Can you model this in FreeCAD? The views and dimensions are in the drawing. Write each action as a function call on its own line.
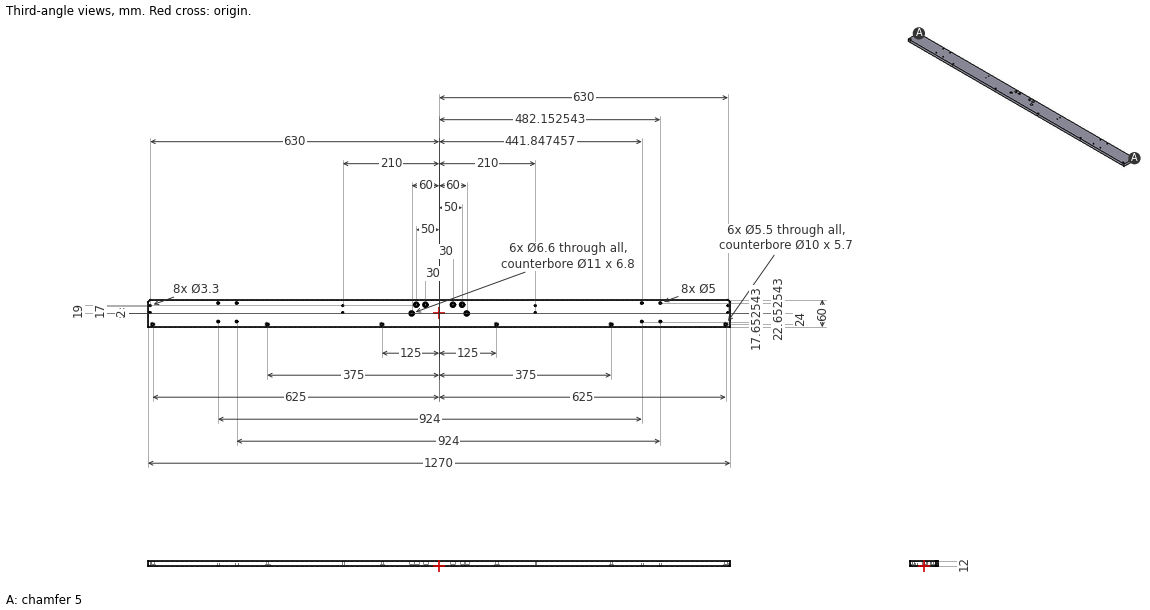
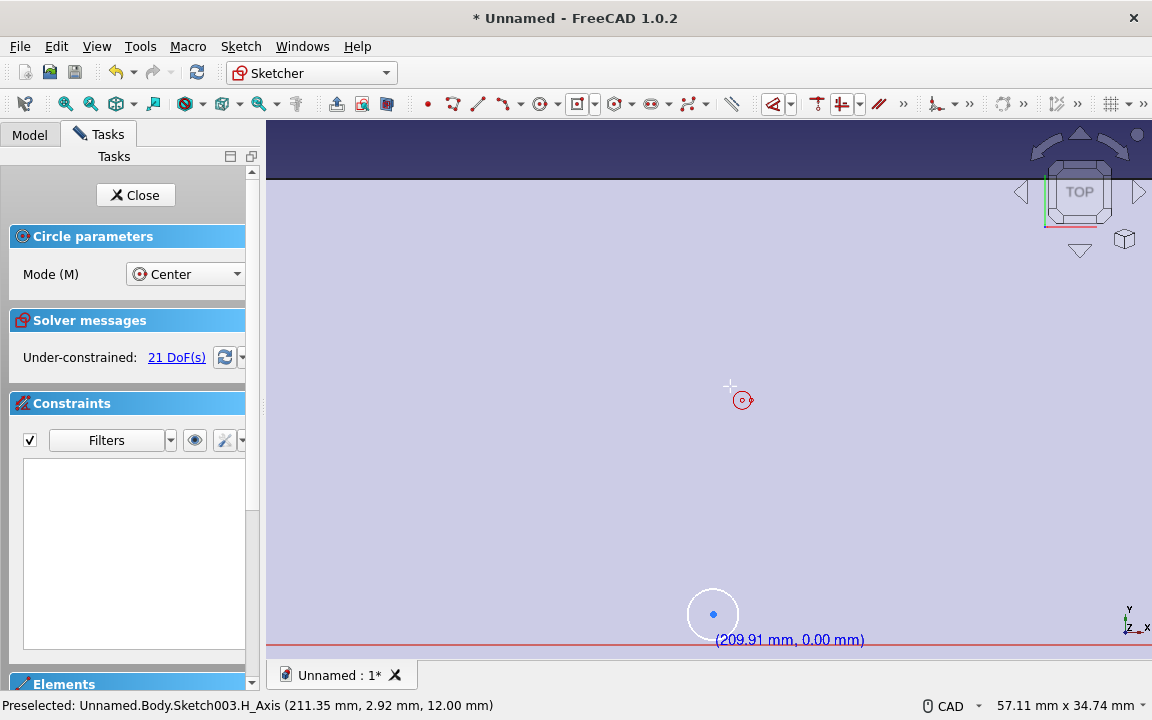
scroll(730, 386, down, 18)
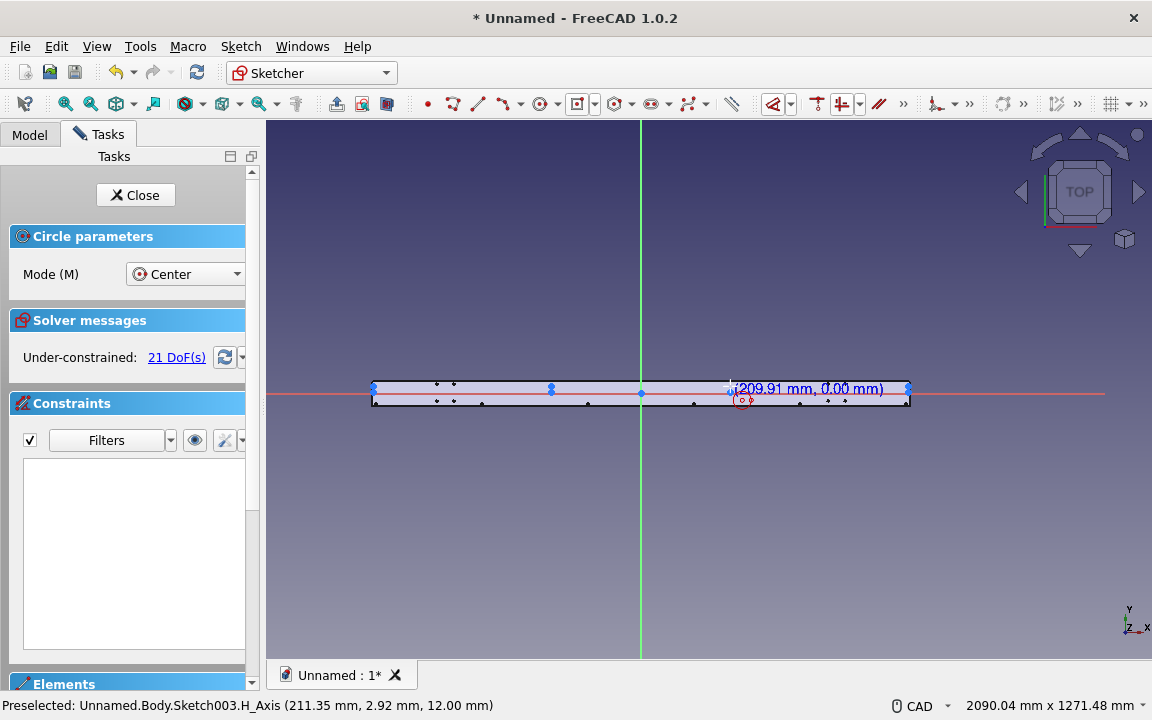
scroll(730, 386, up, 6)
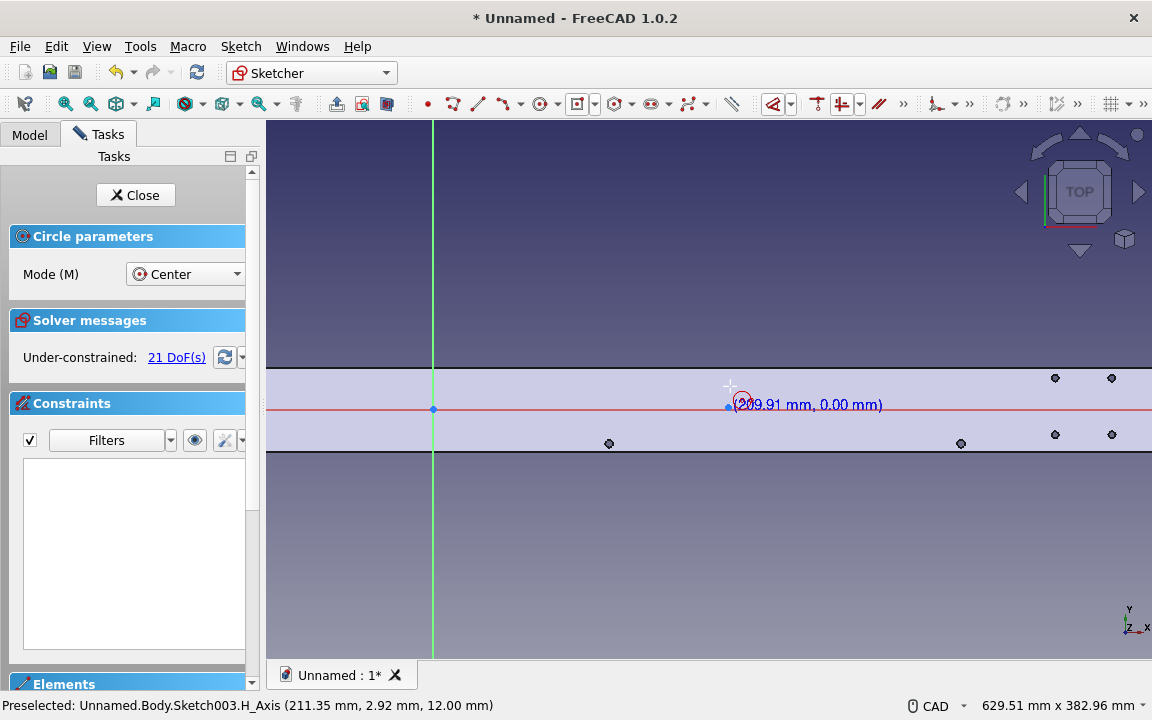
click(729, 386)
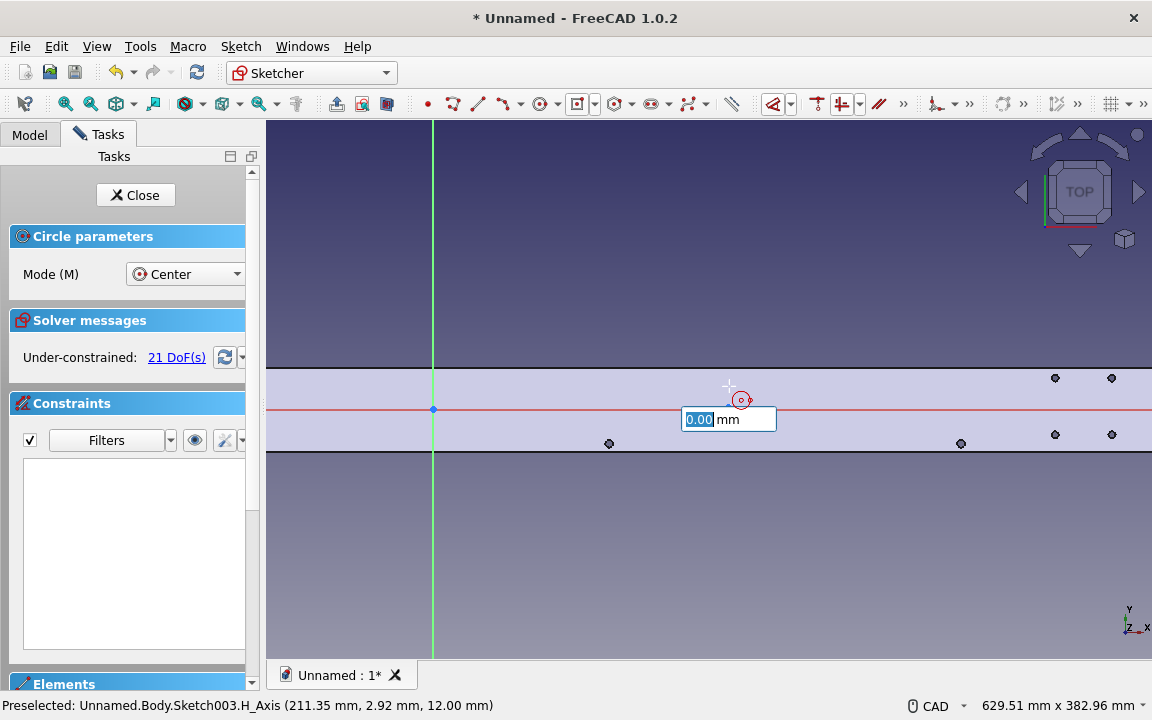
scroll(731, 384, up, 10)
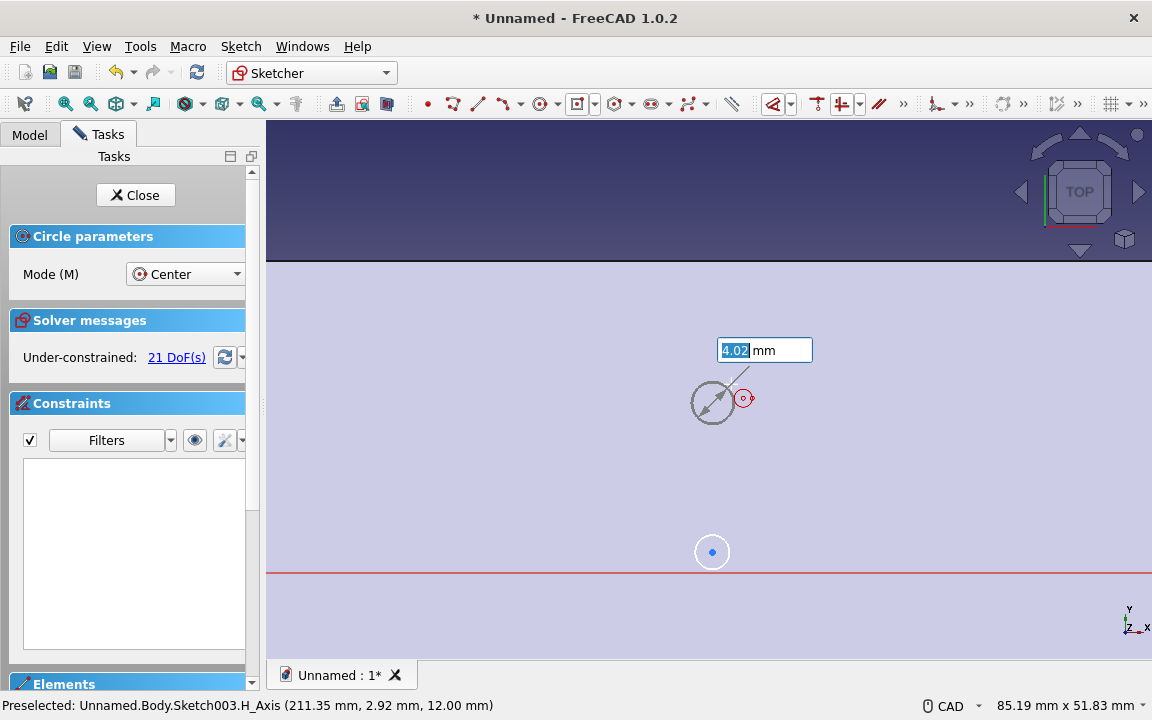
click(724, 384)
key(Escape)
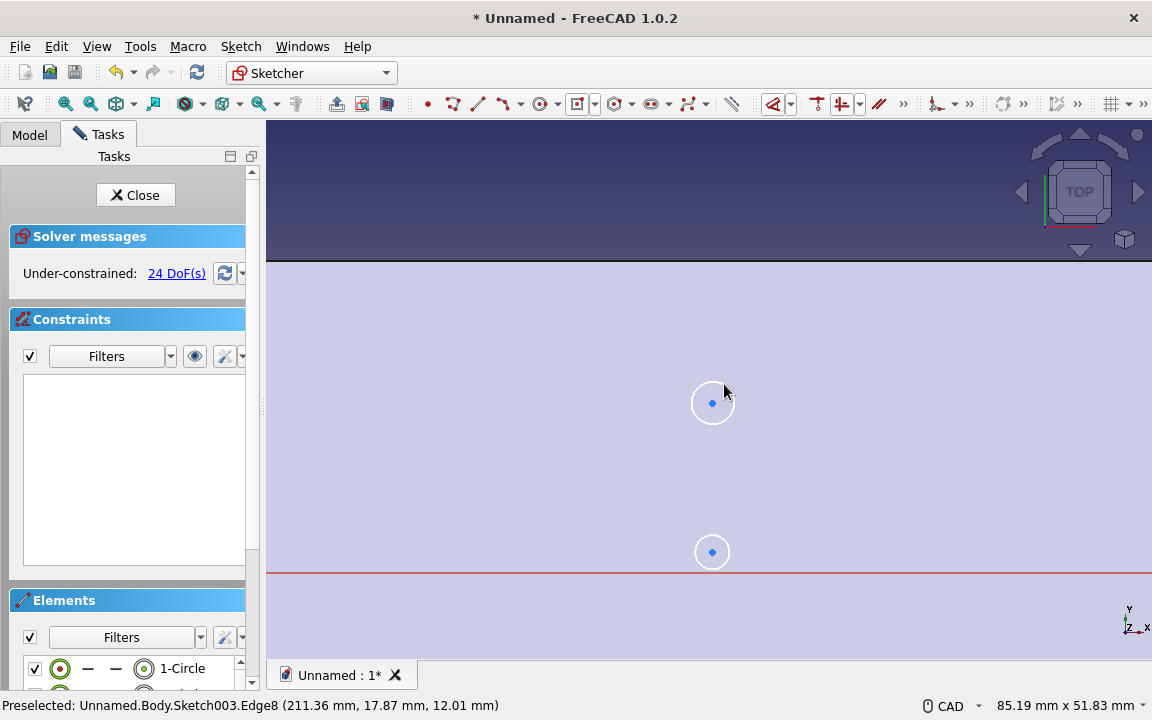
scroll(730, 386, down, 16)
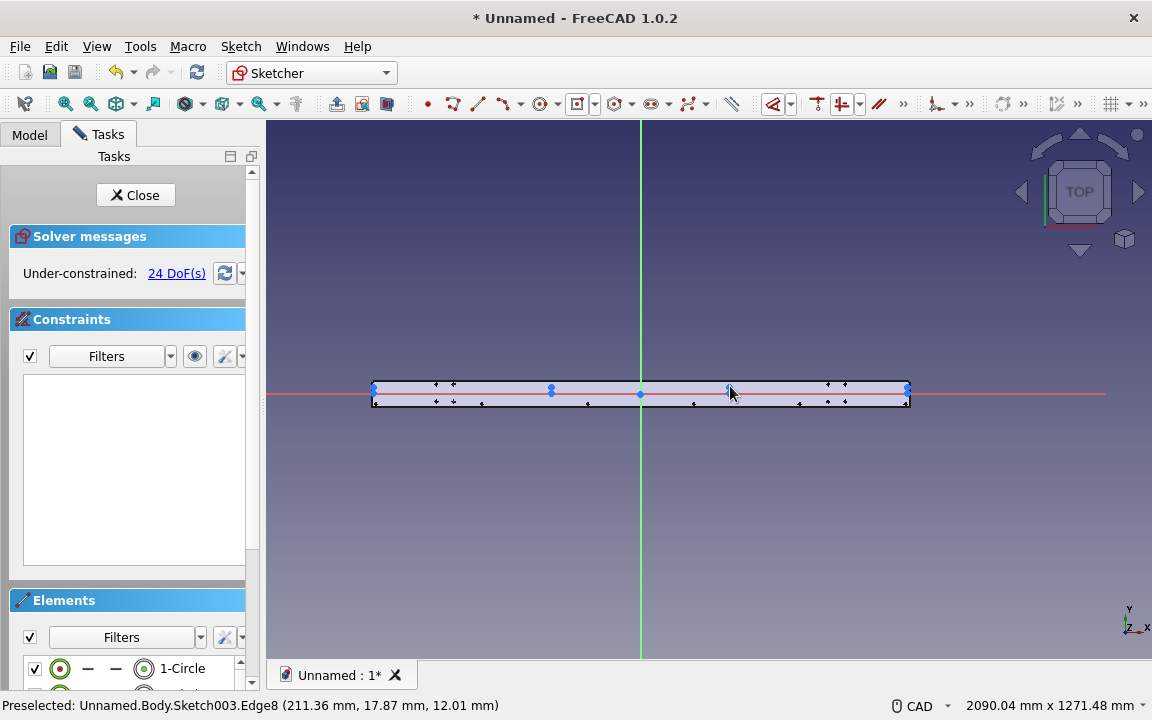
scroll(374, 387, up, 13)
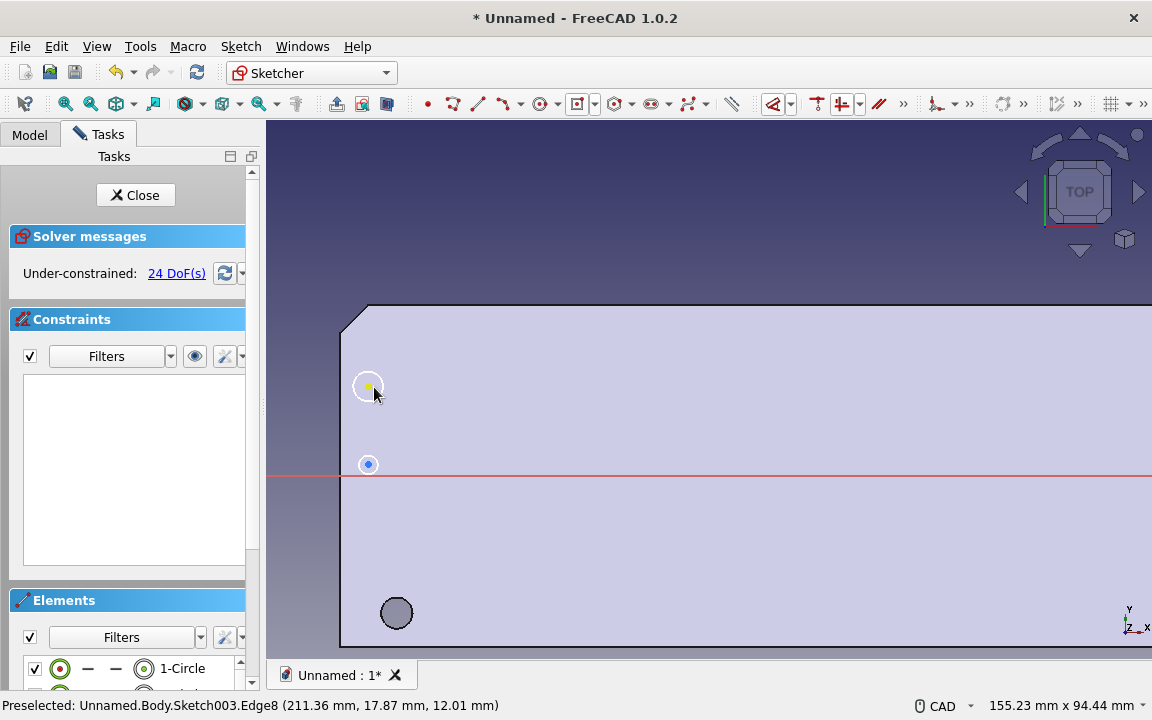
click(379, 376)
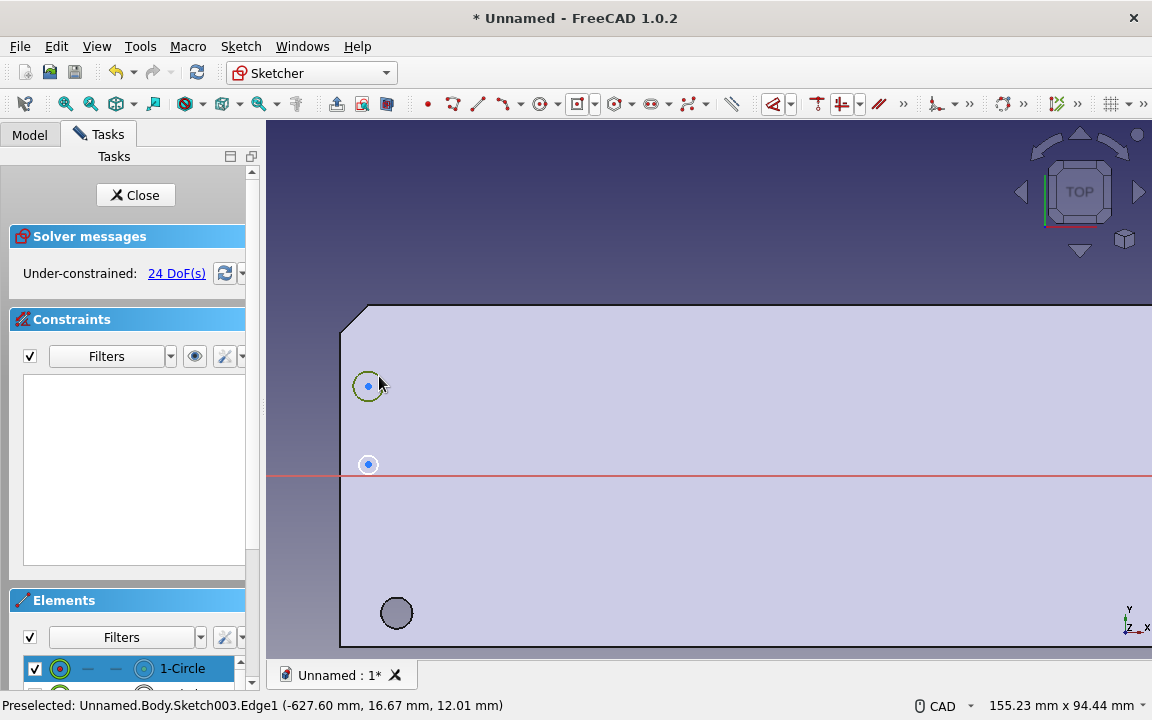
click(375, 458)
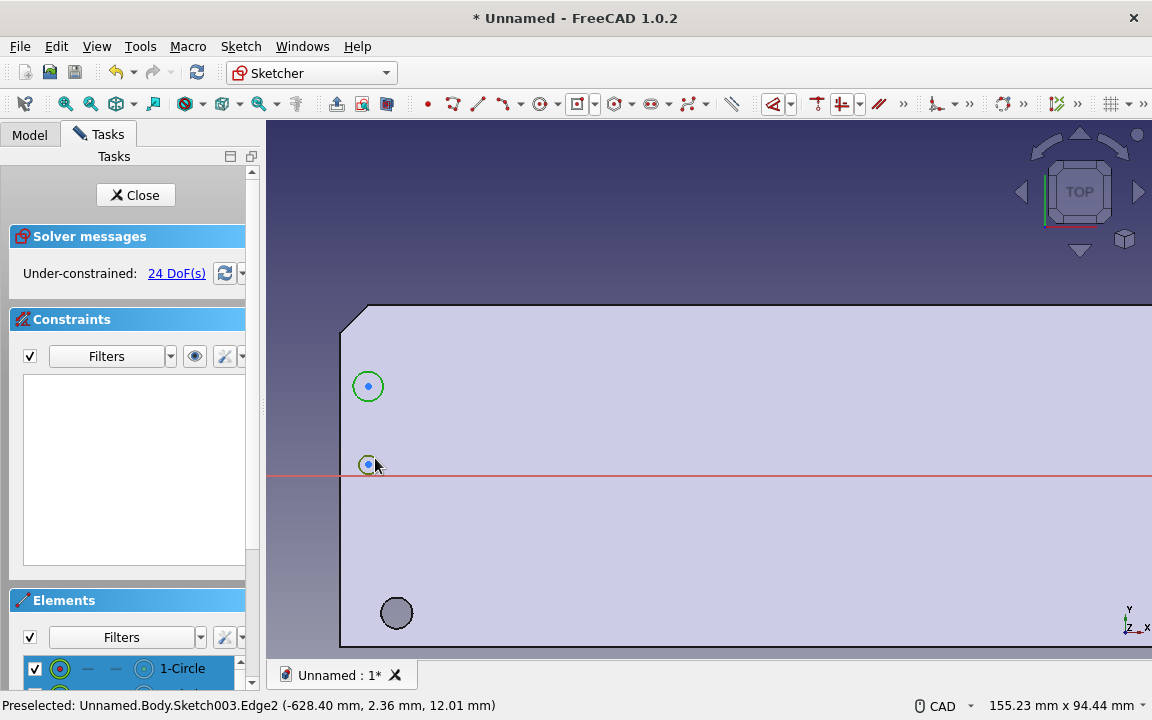
scroll(374, 387, down, 13)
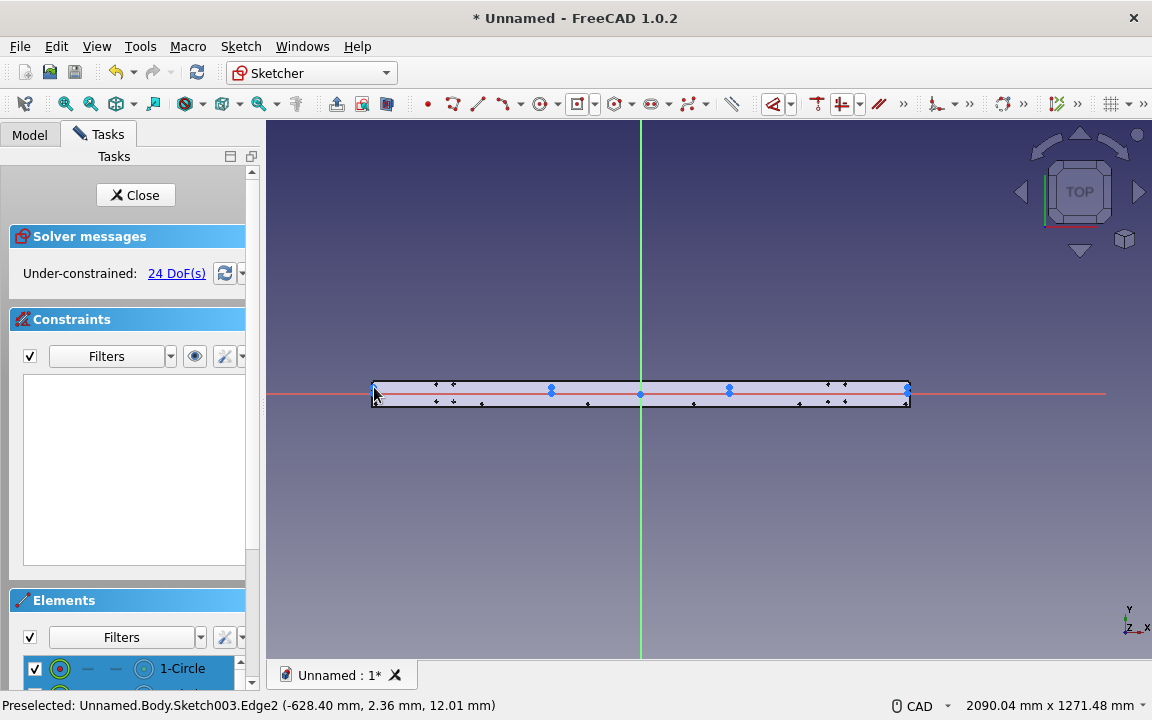
scroll(908, 393, up, 13)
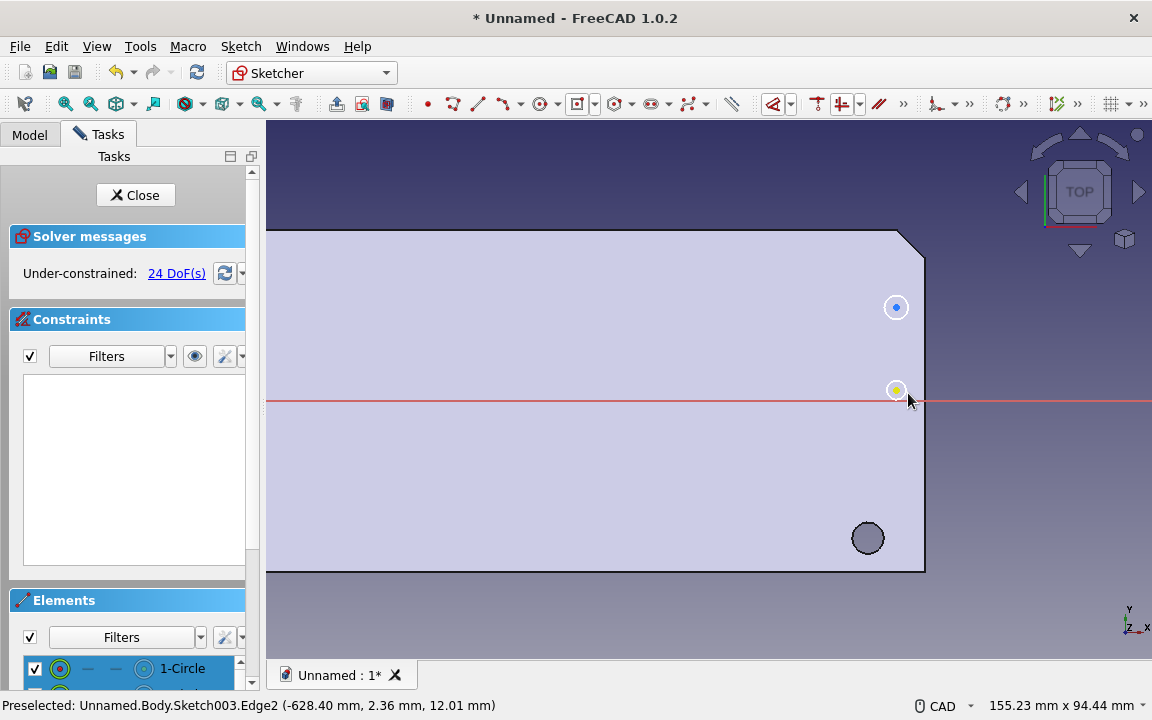
click(903, 384)